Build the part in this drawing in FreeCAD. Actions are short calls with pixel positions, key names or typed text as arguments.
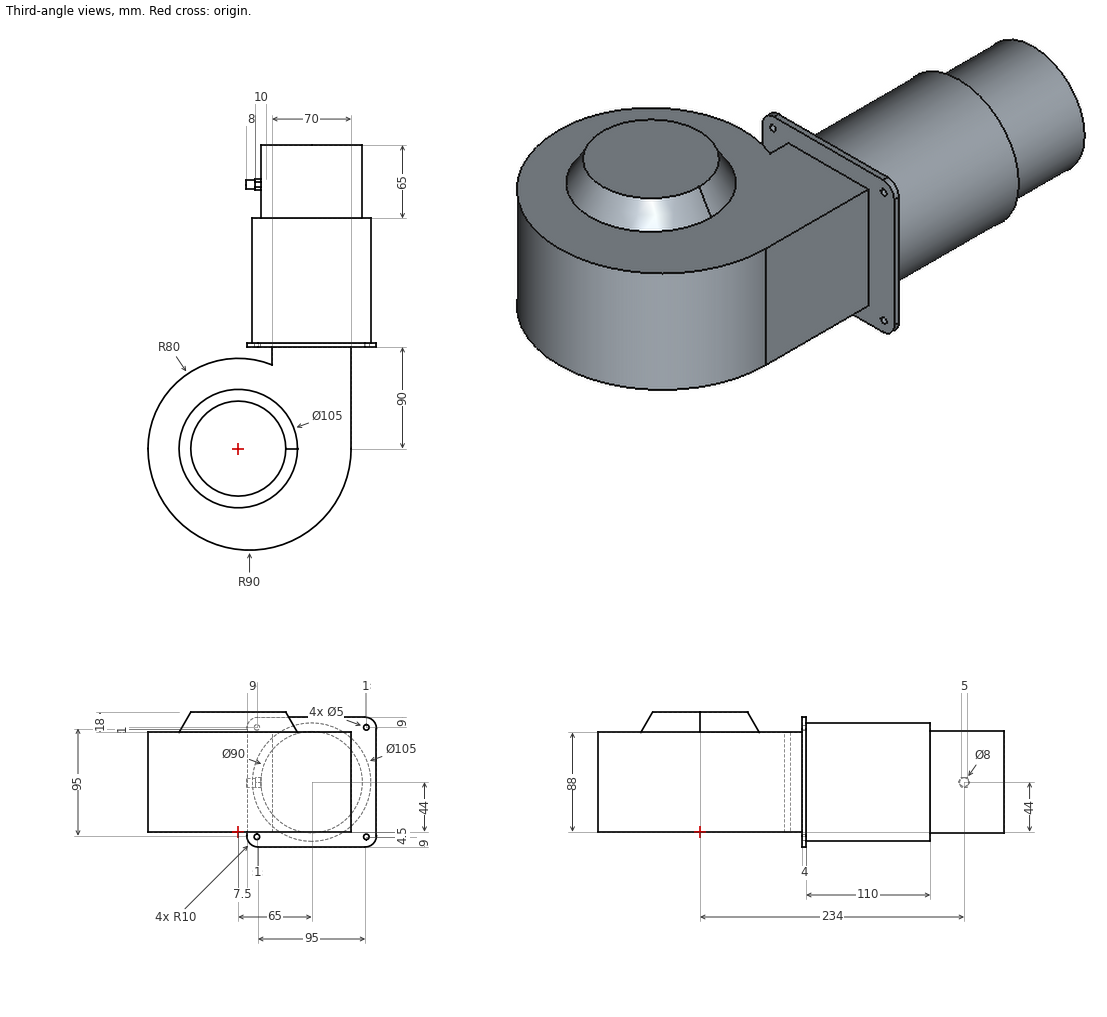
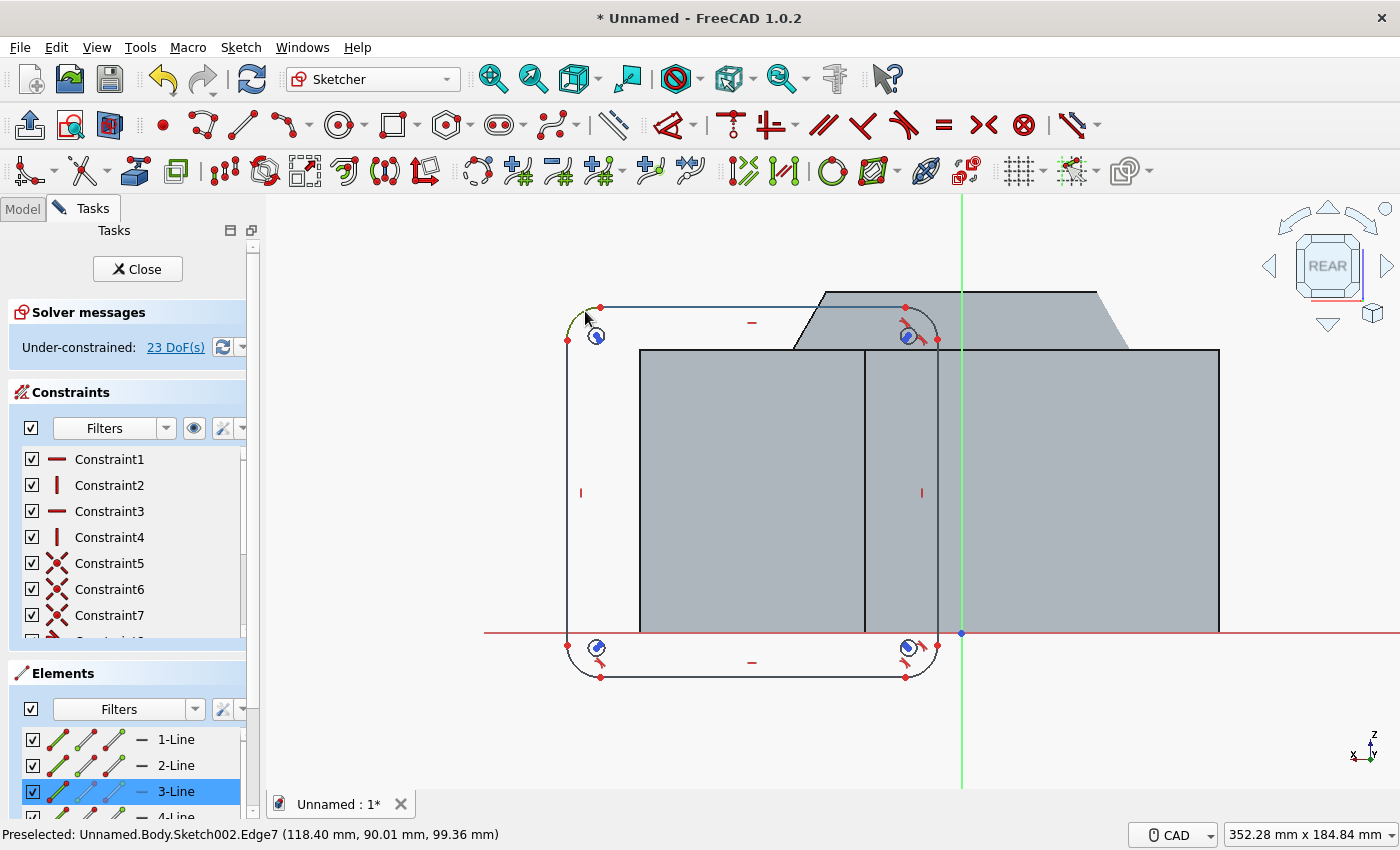
click(904, 126)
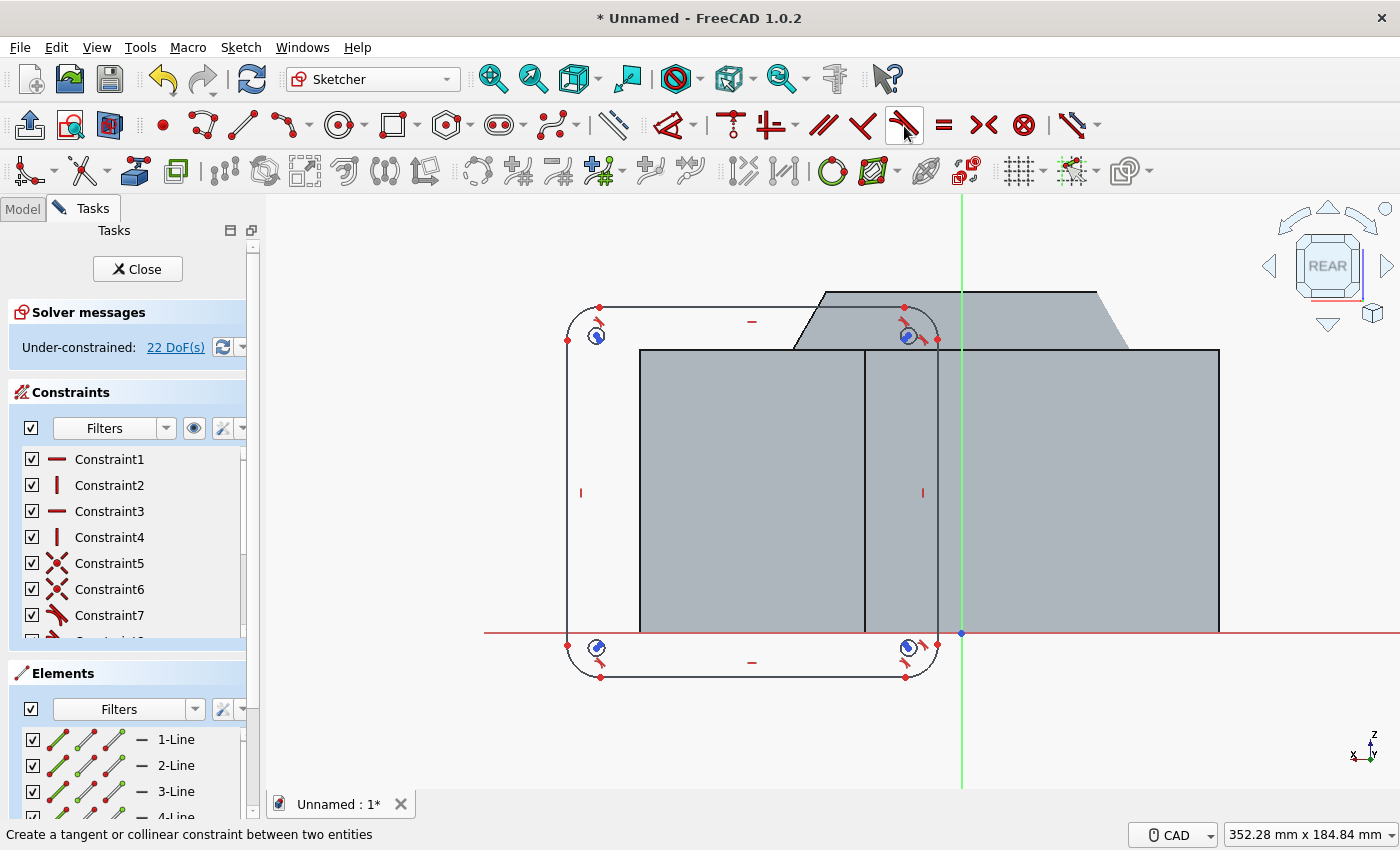
click(567, 432)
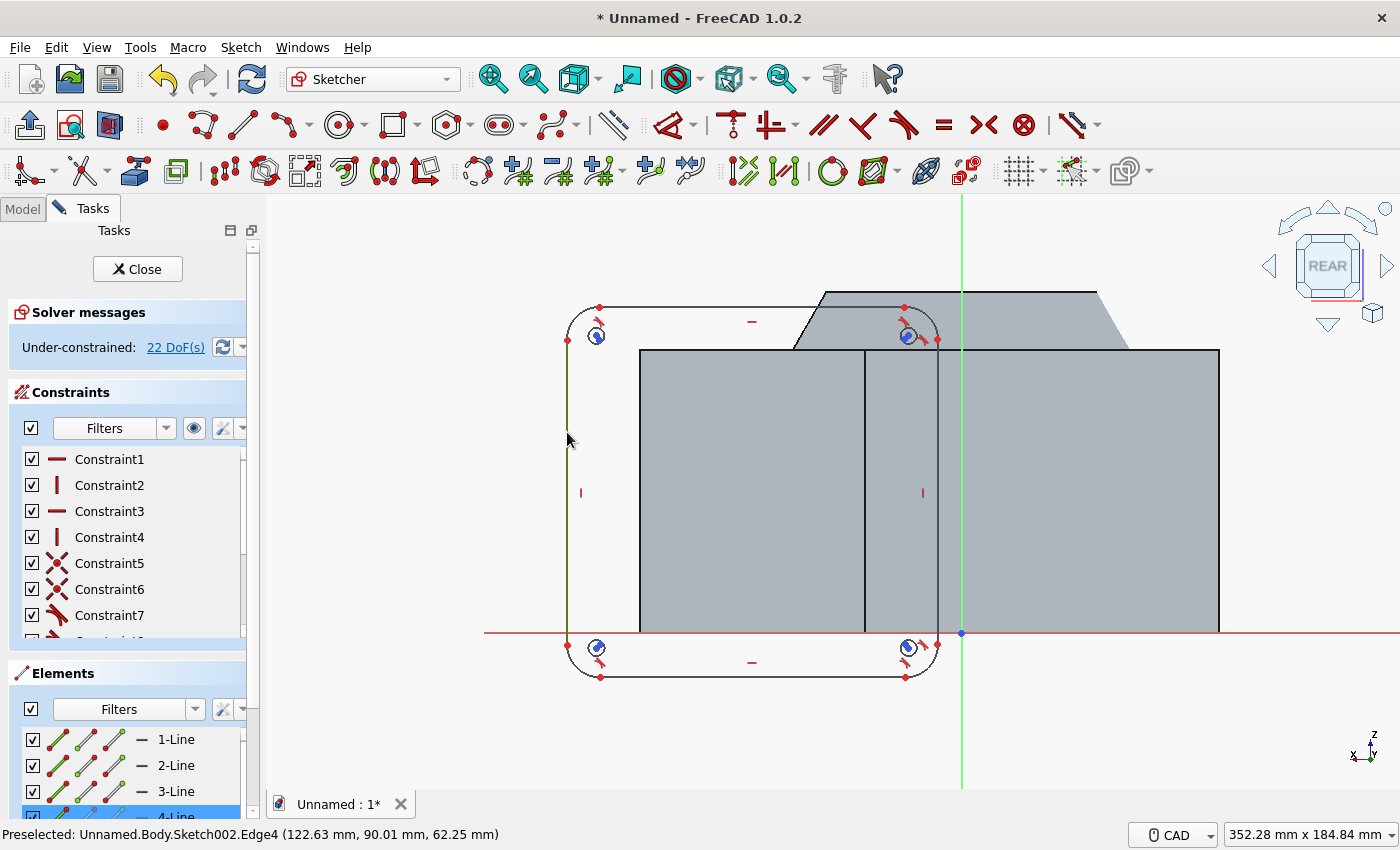
click(585, 311)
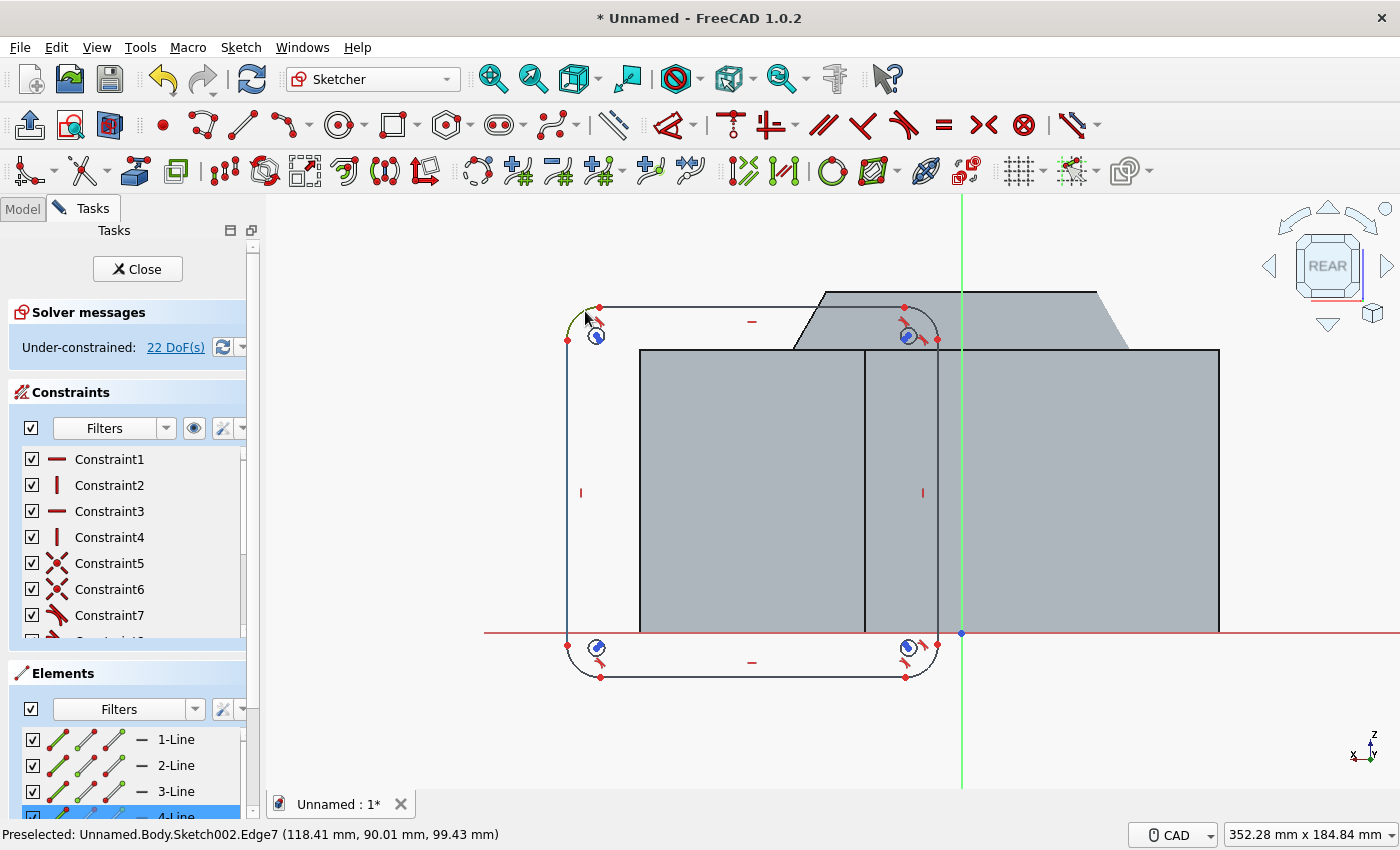
key(t)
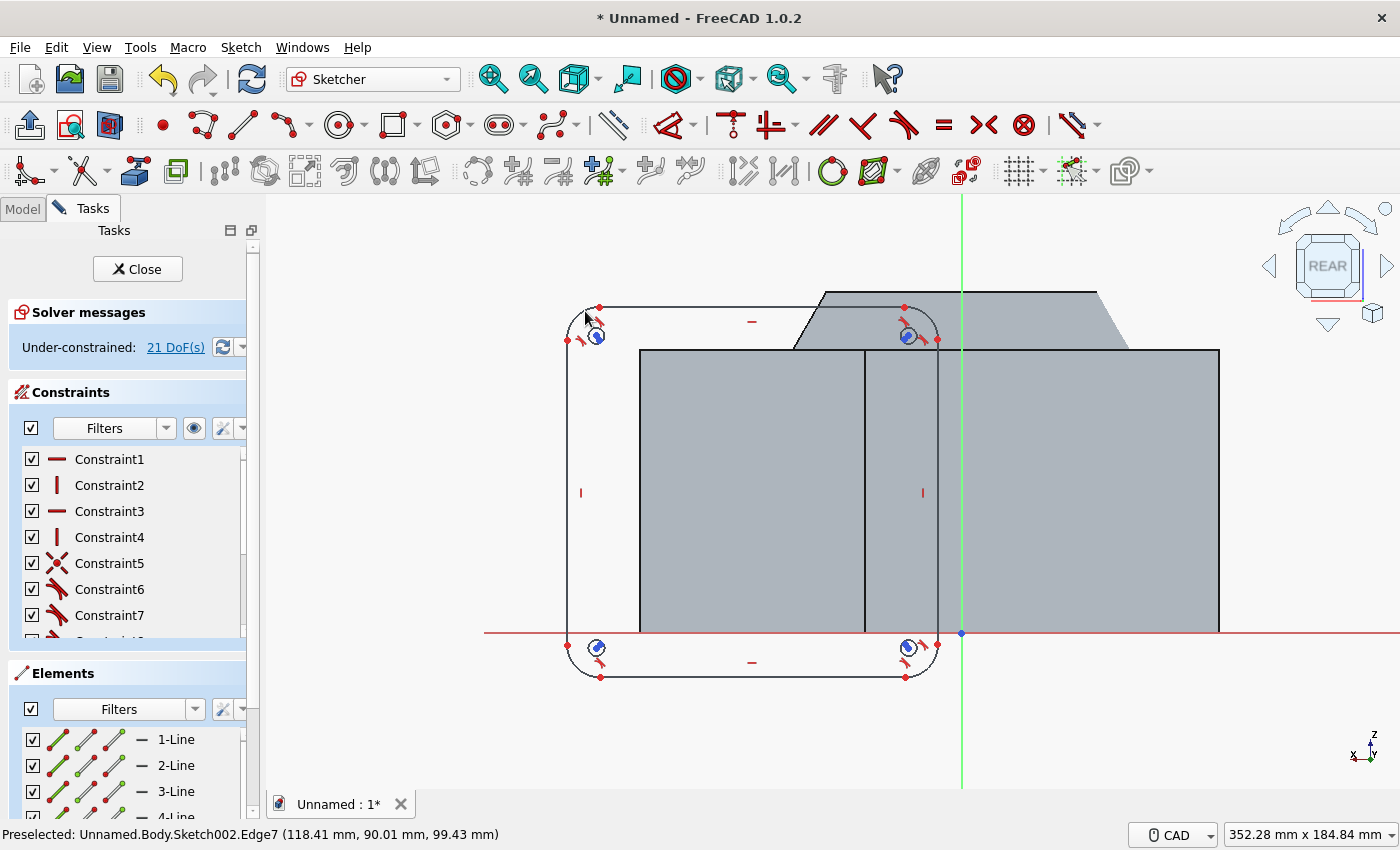
click(567, 432)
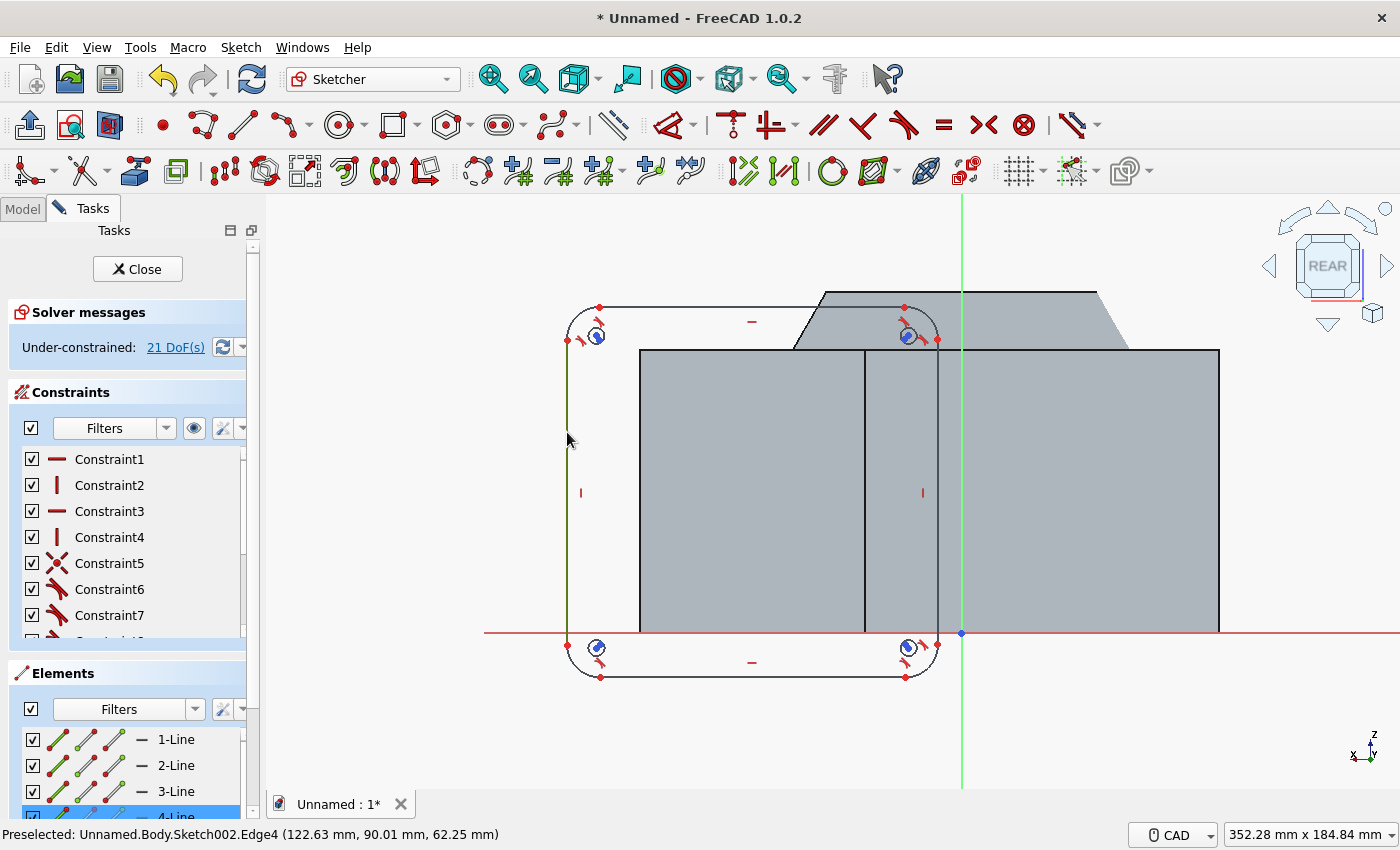
click(571, 660)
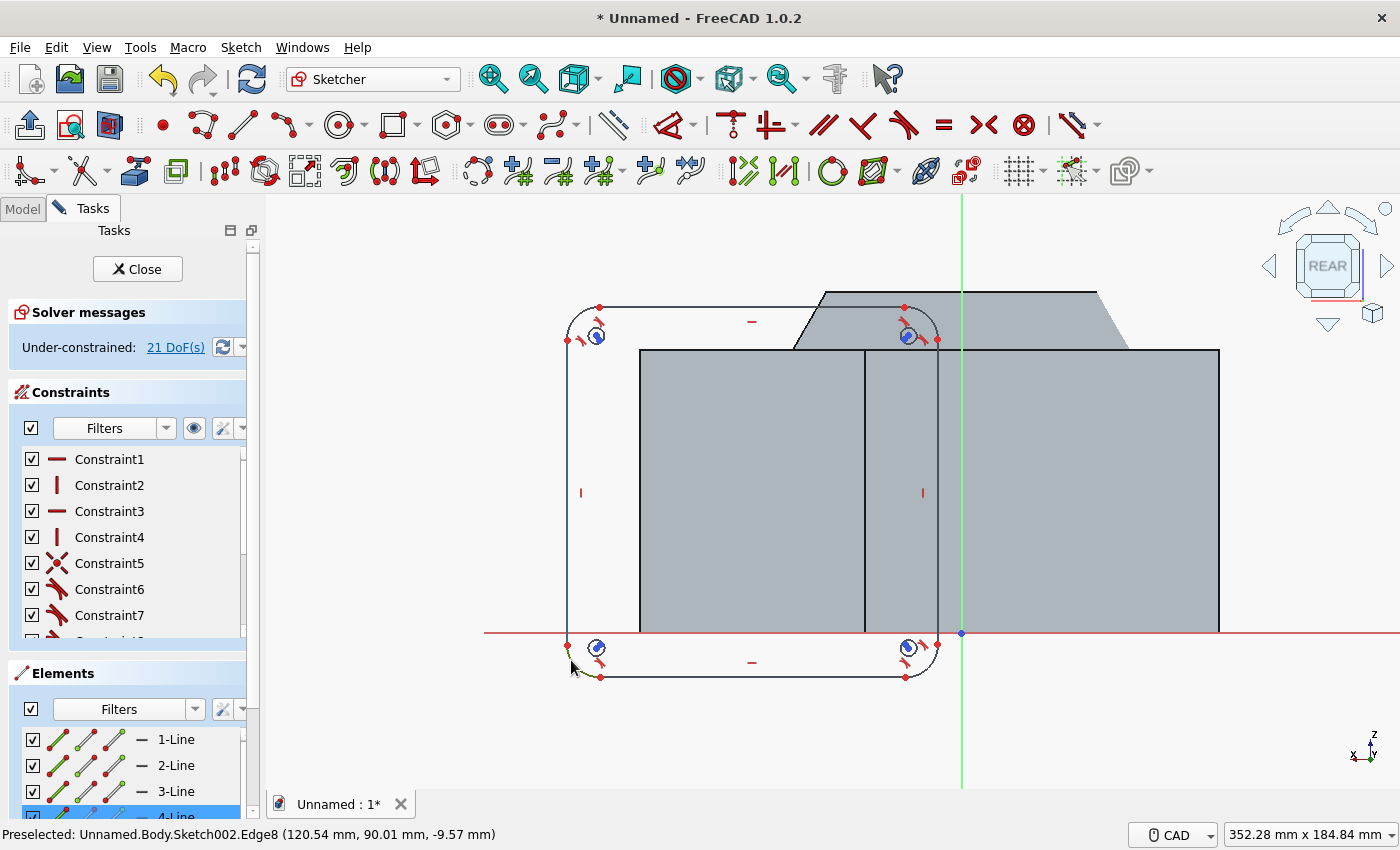
click(904, 126)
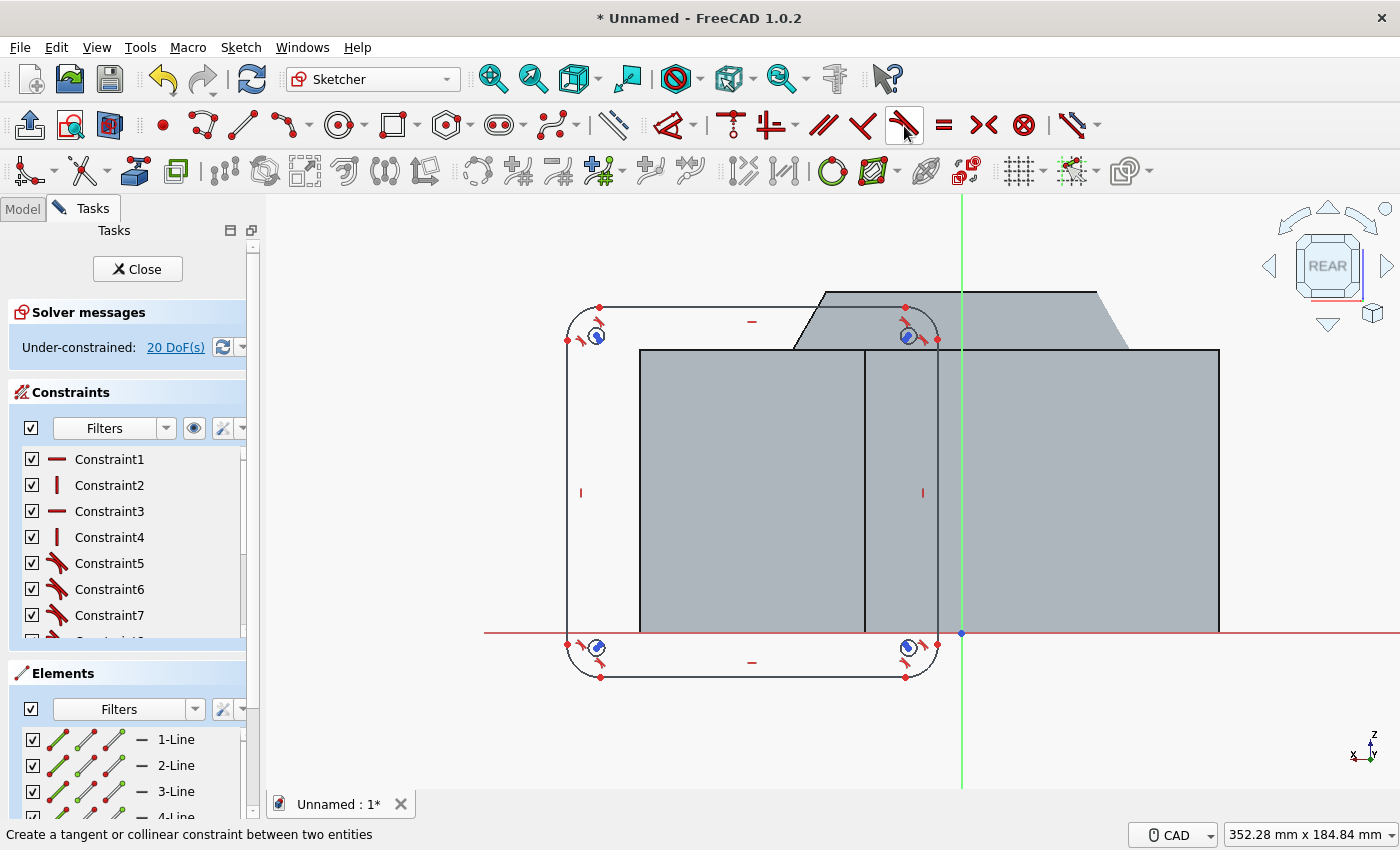
click(920, 674)